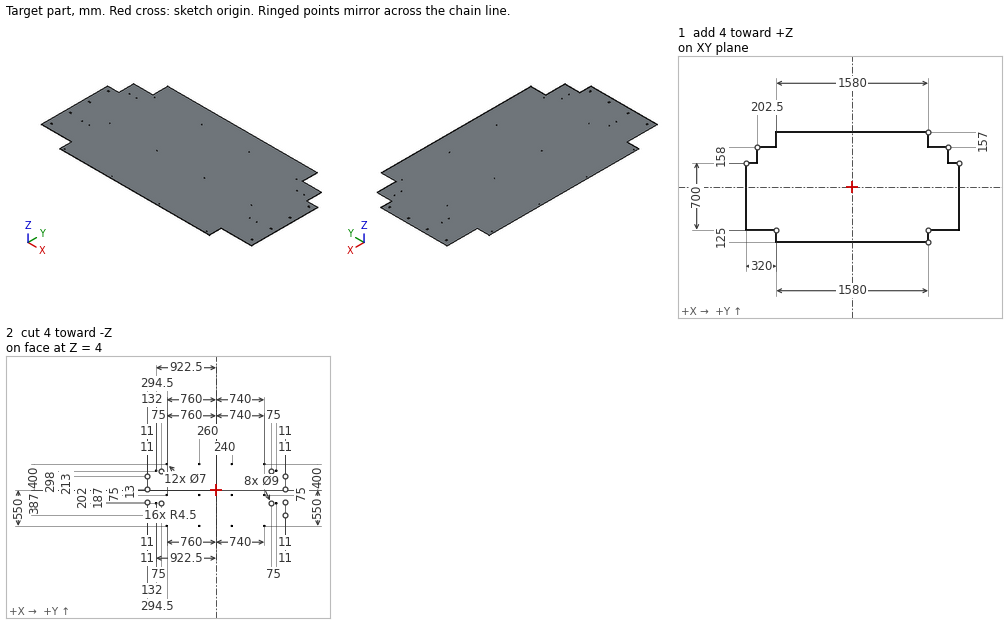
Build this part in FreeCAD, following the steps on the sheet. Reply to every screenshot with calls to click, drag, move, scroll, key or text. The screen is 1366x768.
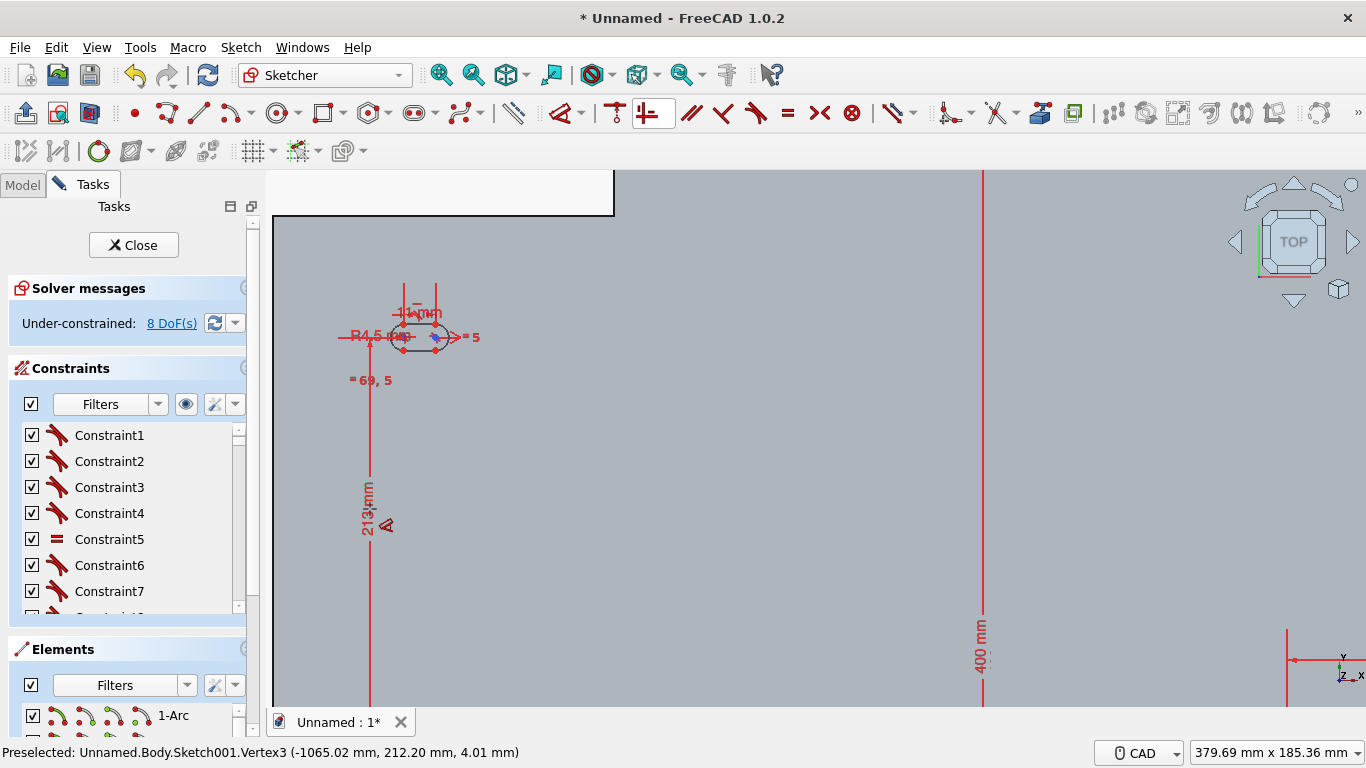
scroll(406, 347, down, 11)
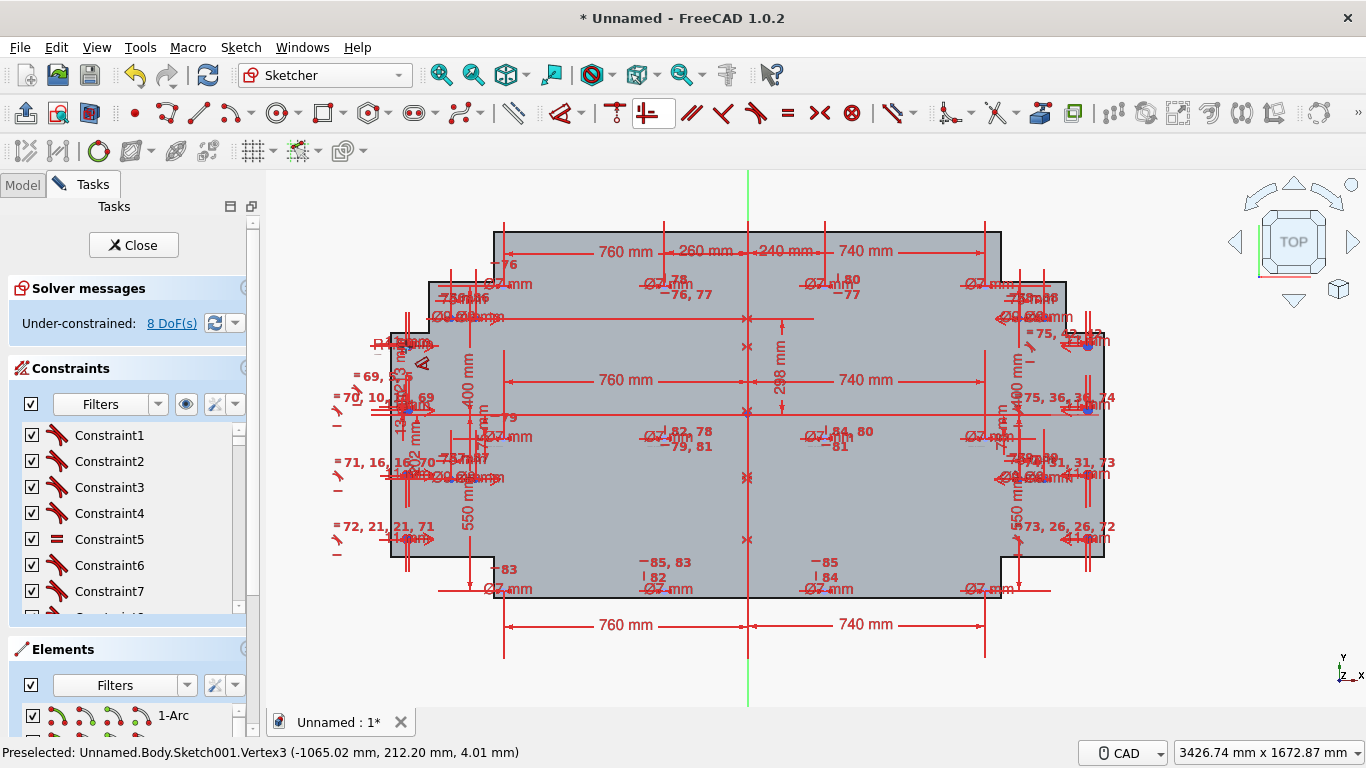
scroll(406, 475, up, 11)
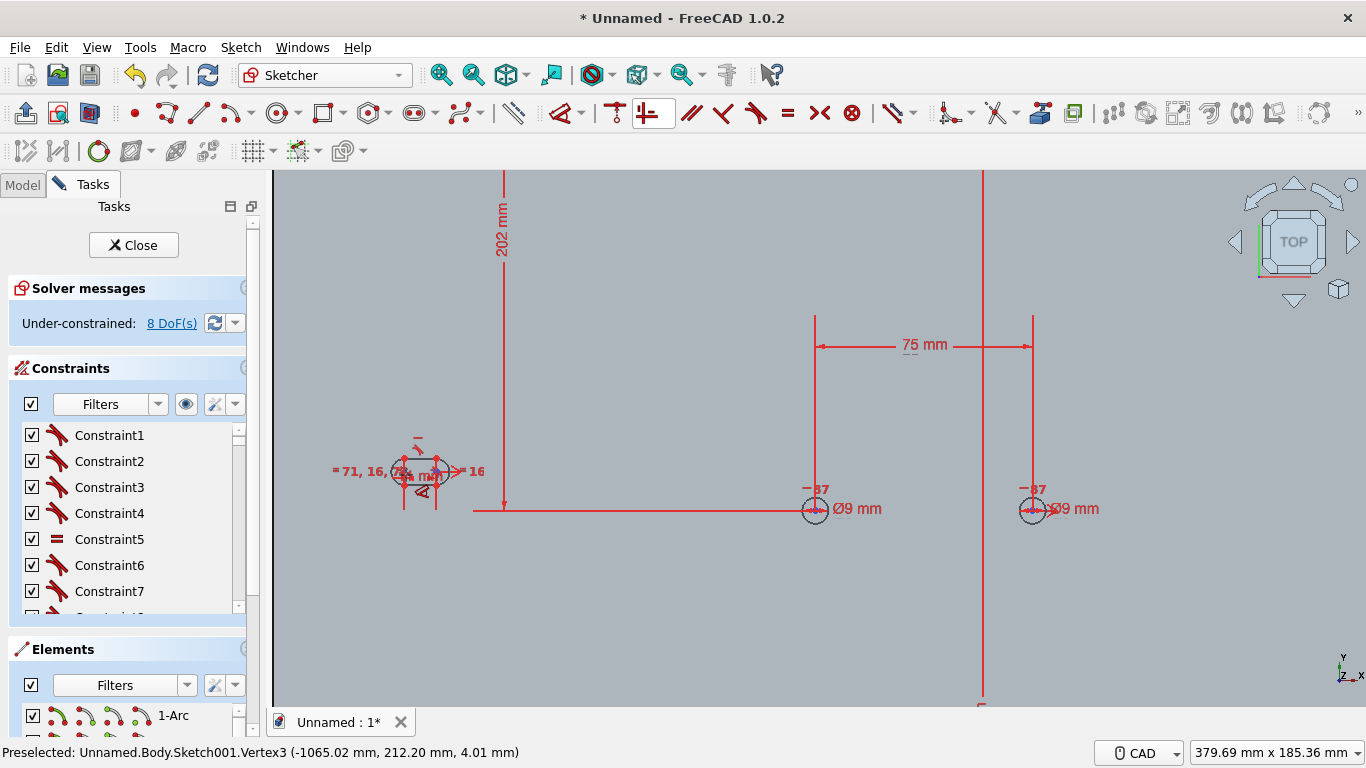
click(404, 472)
click(370, 335)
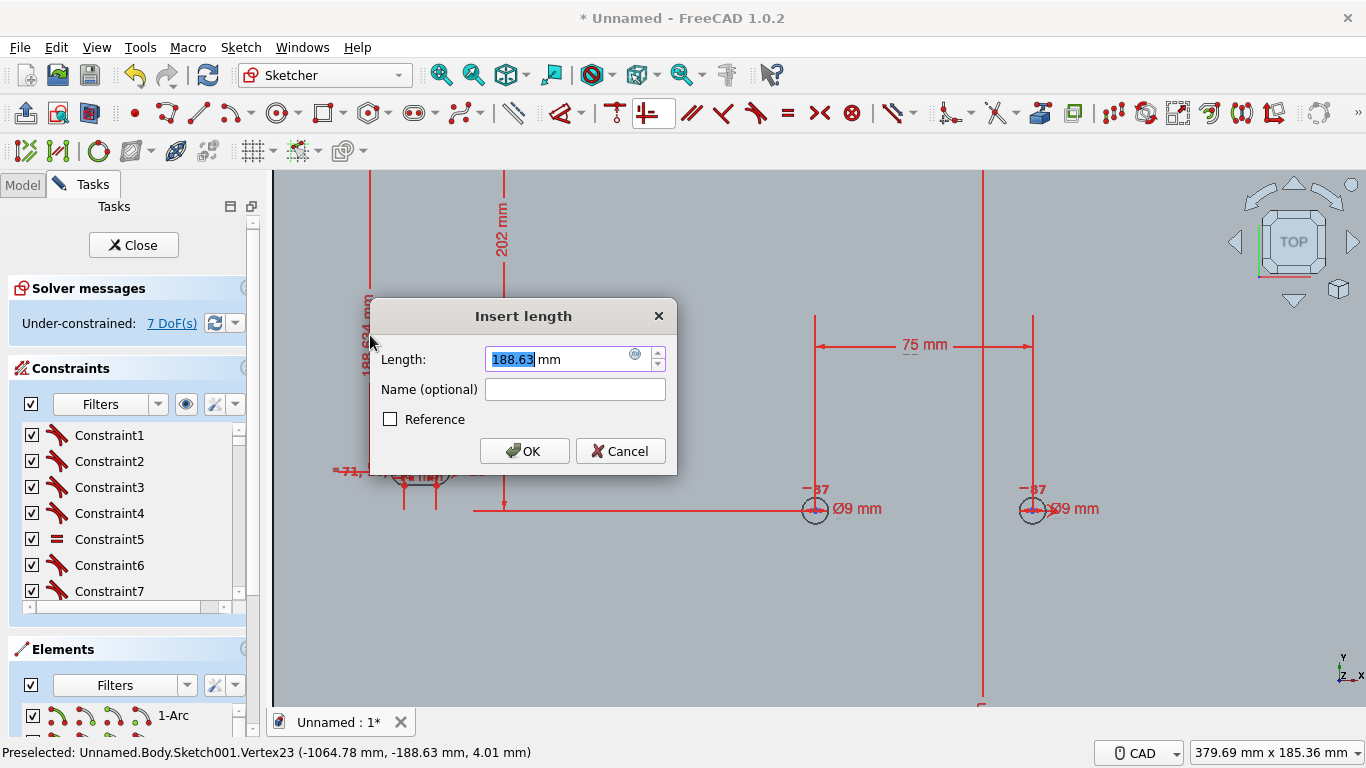
text(187)
key(Return)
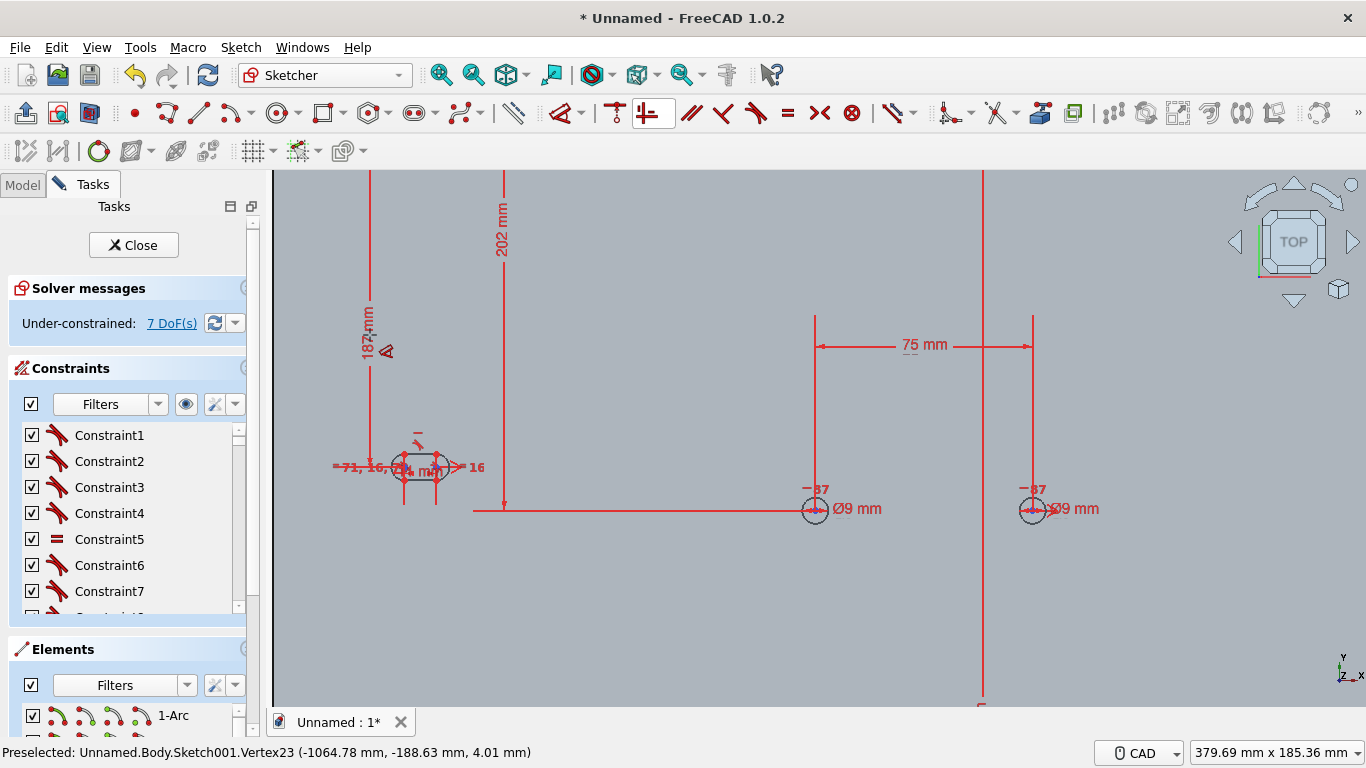
scroll(406, 475, down, 11)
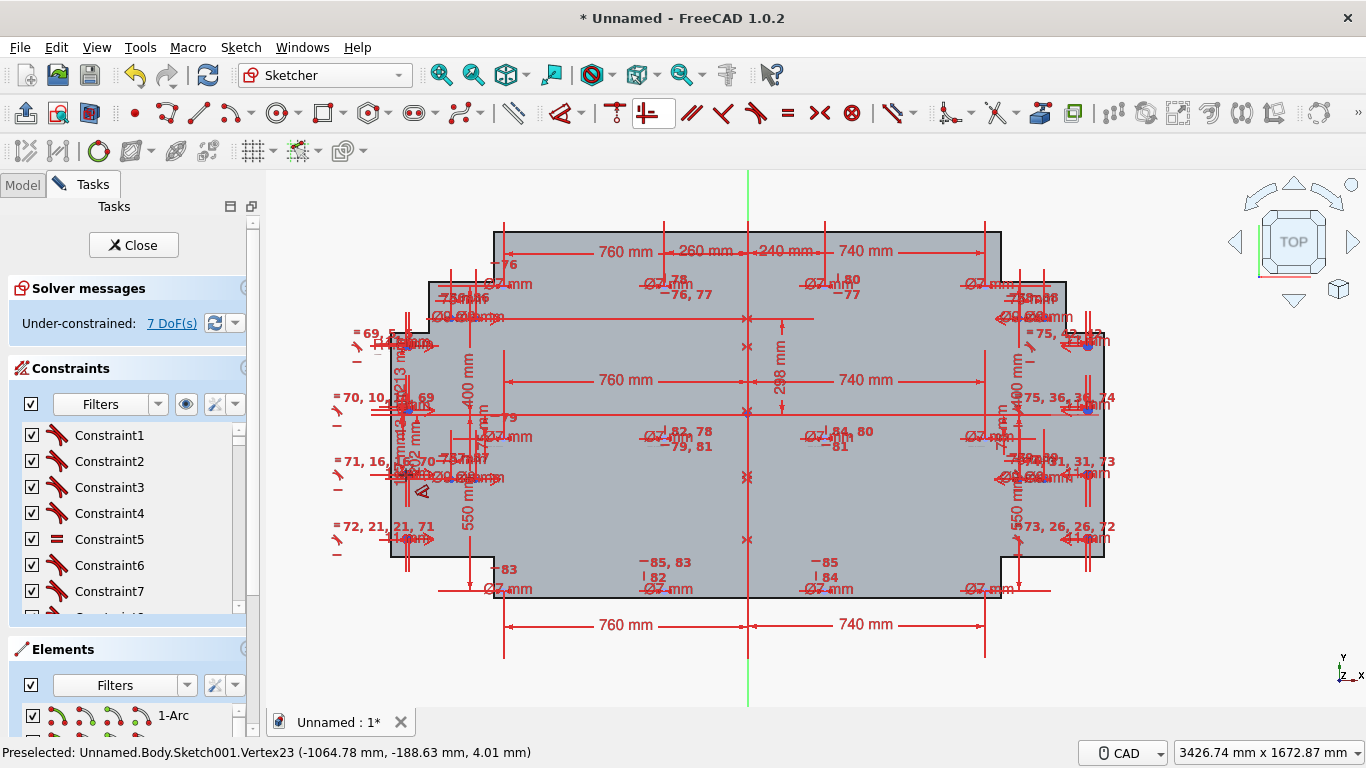
scroll(406, 539, up, 11)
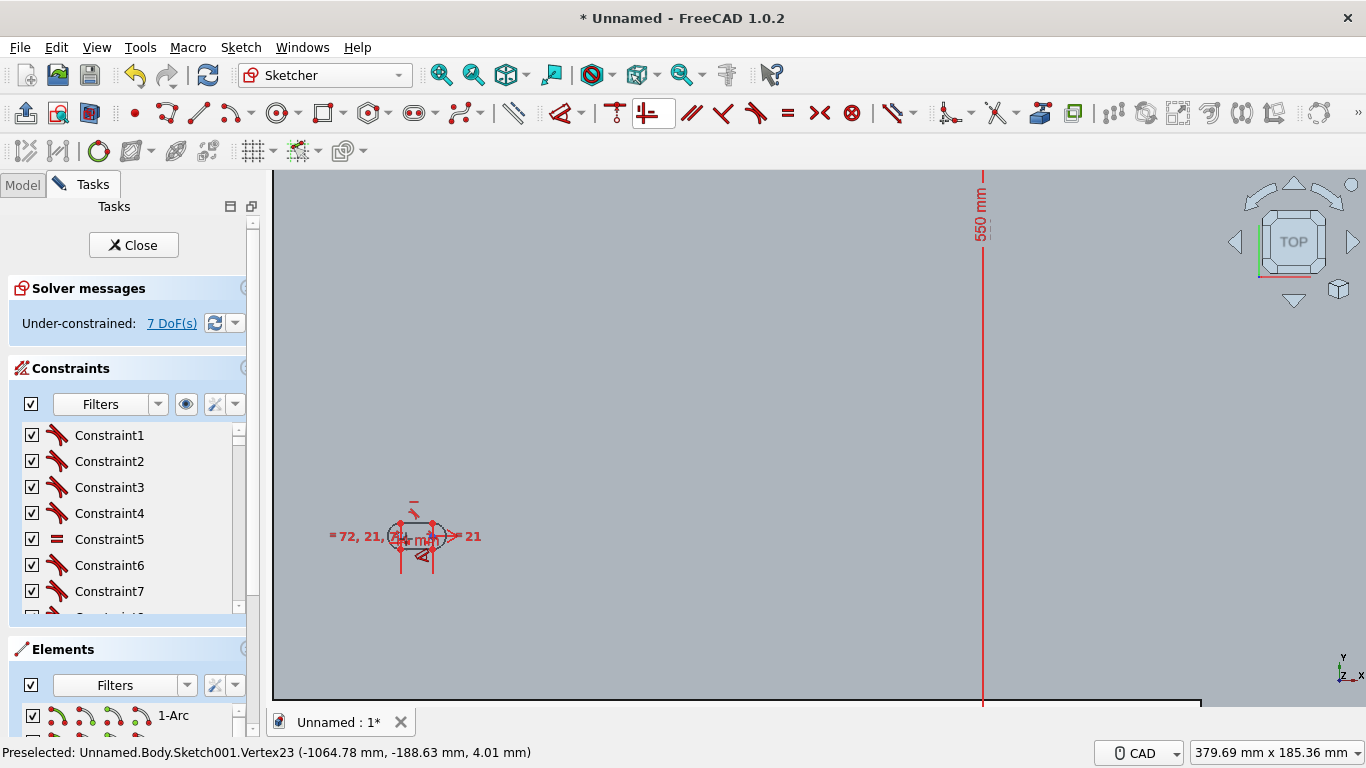
click(401, 536)
click(367, 367)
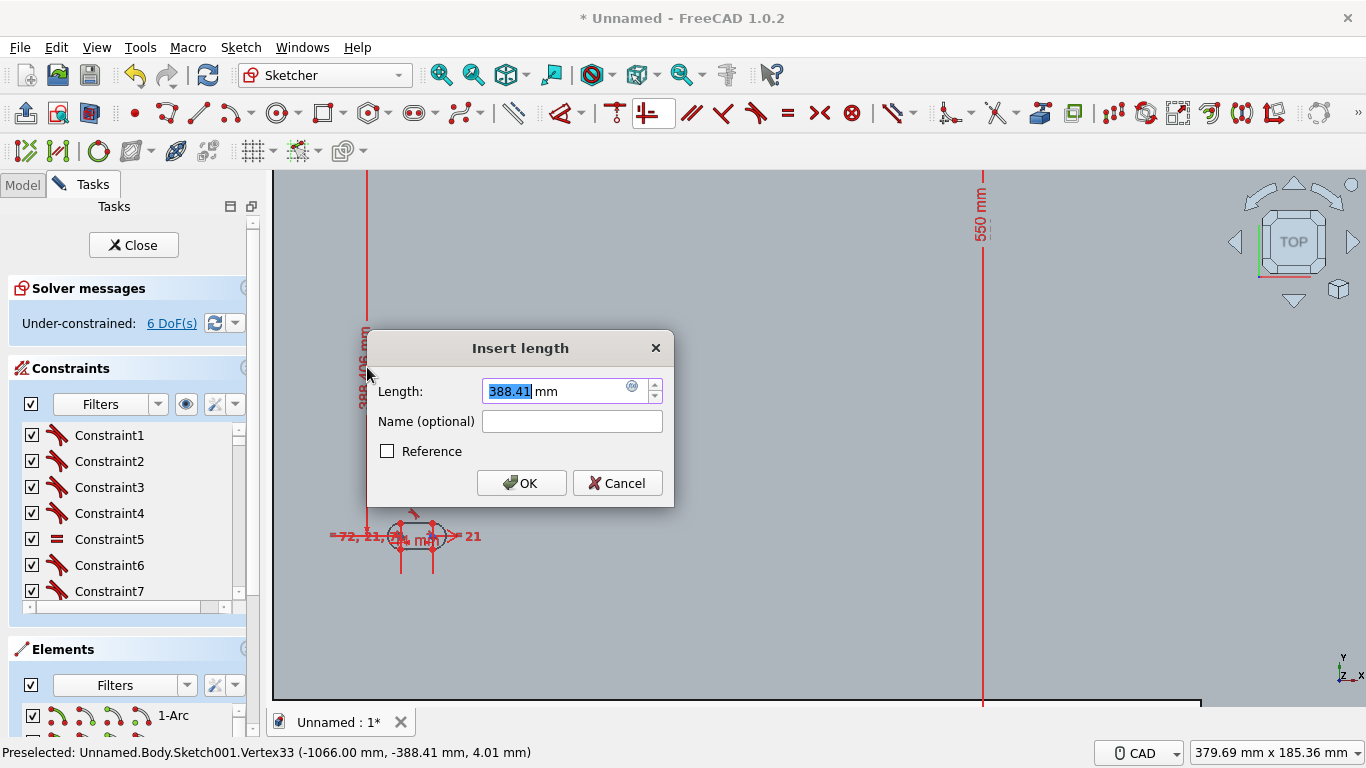
text(387)
key(Return)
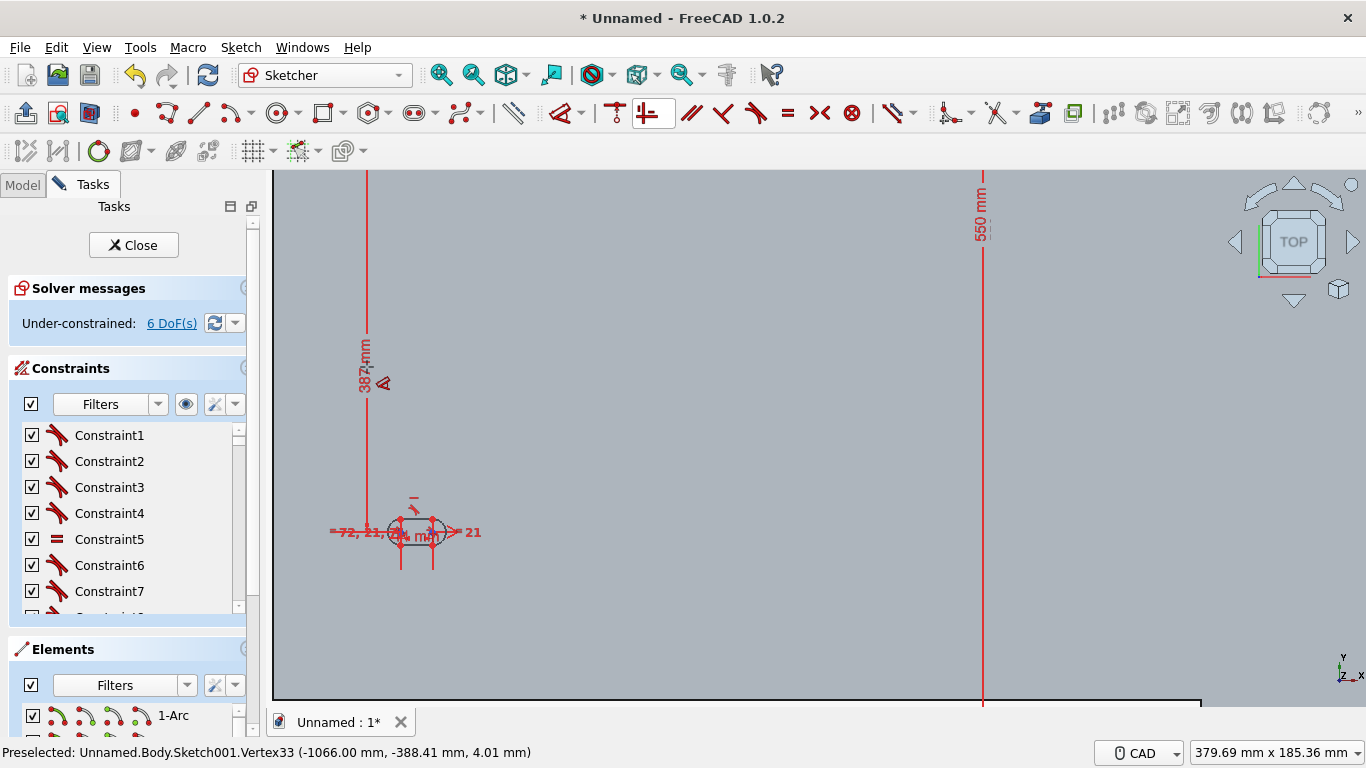
scroll(406, 539, down, 11)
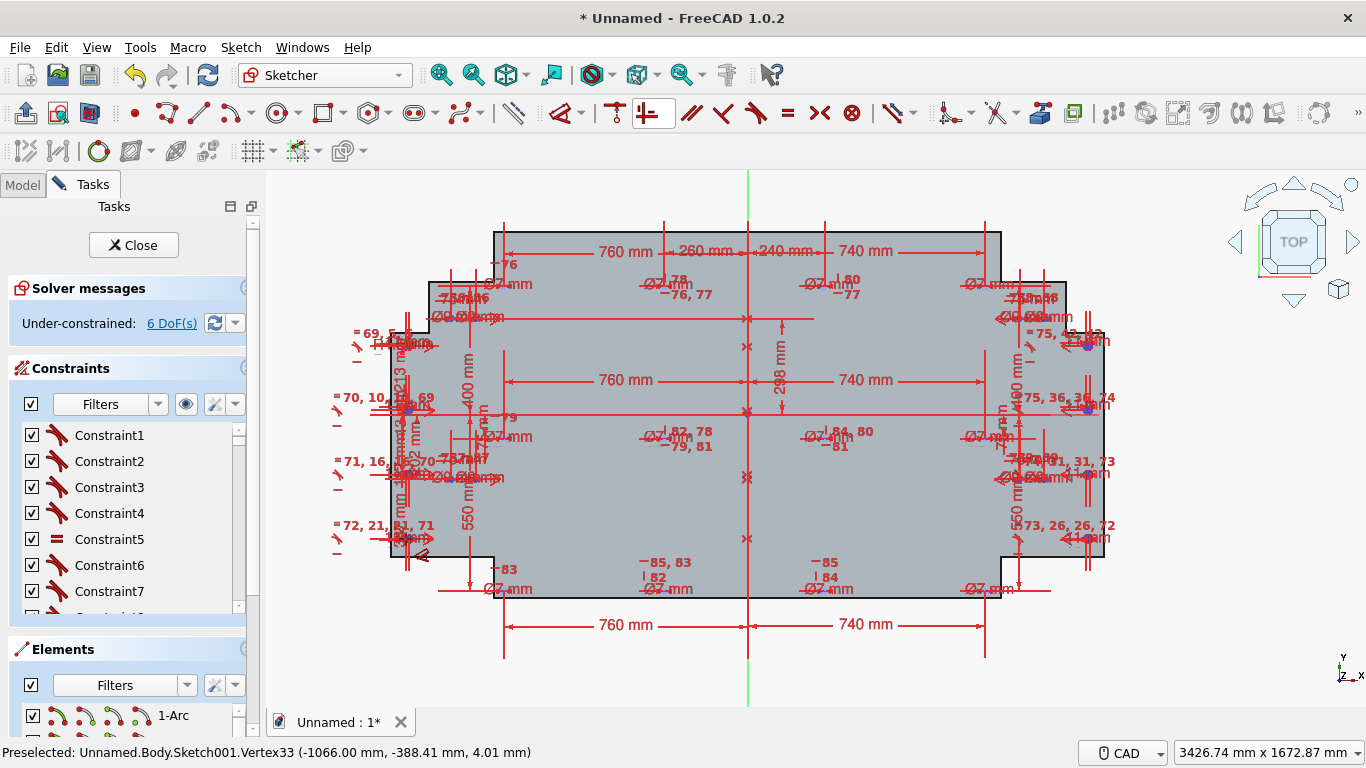
scroll(409, 345, up, 11)